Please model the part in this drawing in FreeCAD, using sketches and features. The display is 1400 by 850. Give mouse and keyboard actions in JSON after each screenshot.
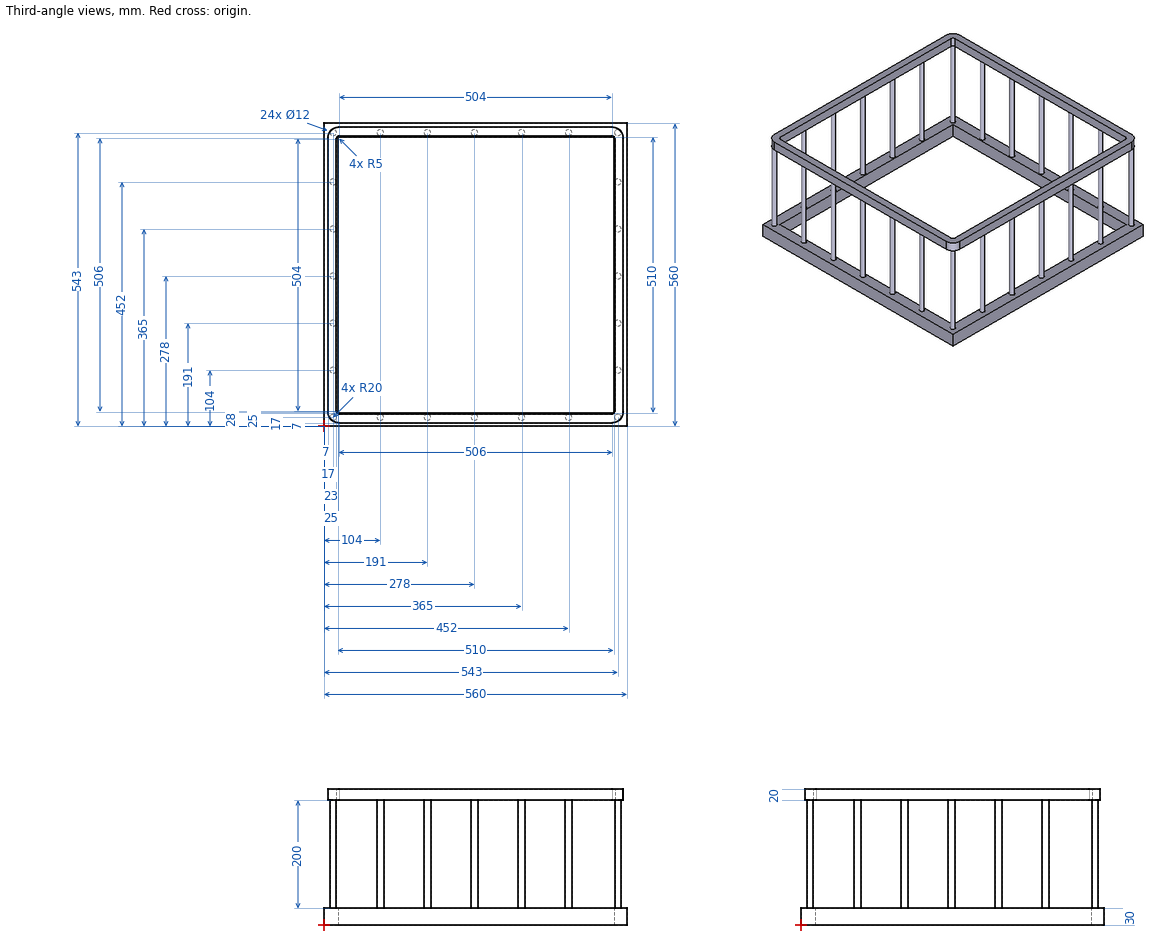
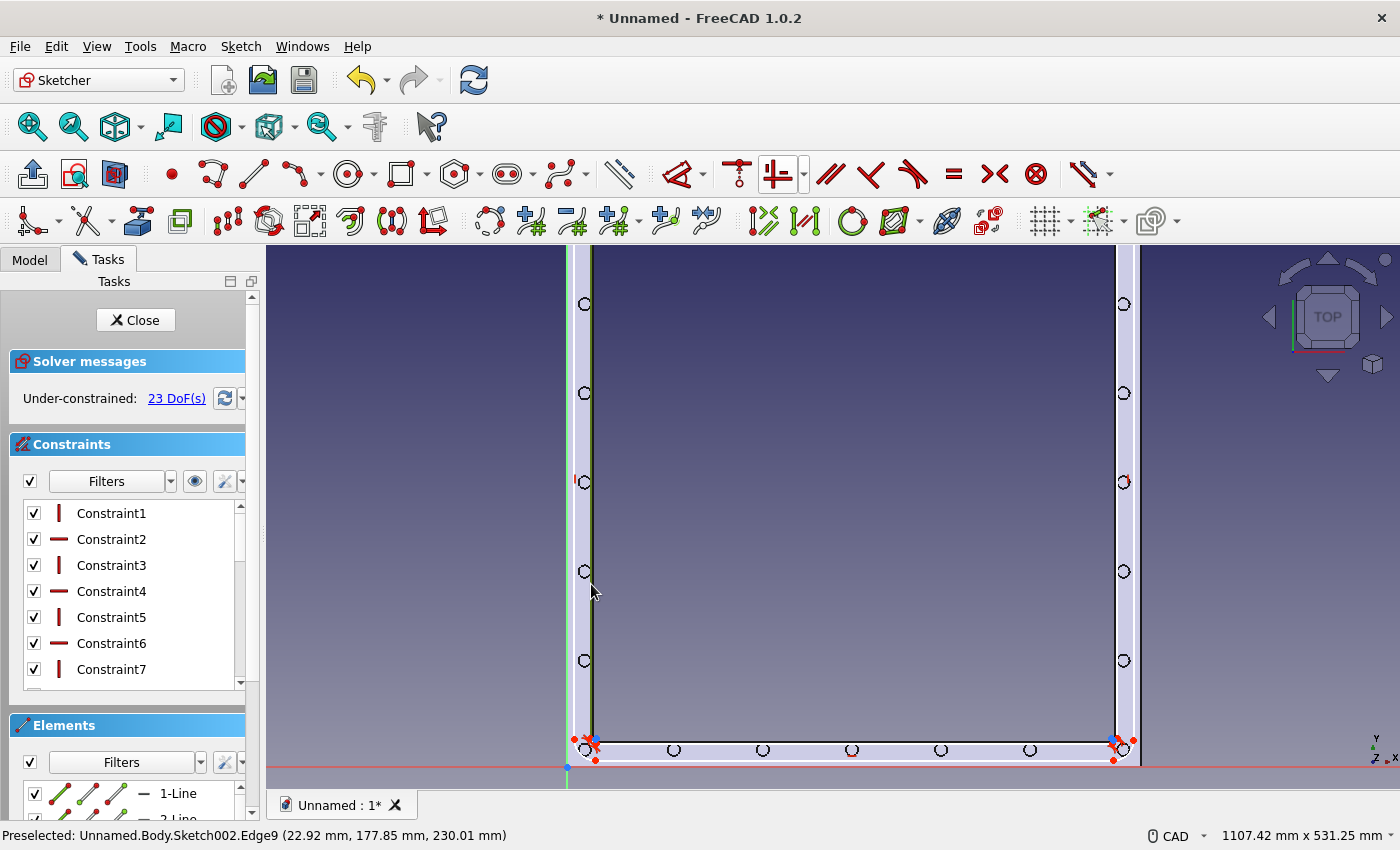
{"action": "scroll", "coordinate": [592, 742], "scroll_direction": "up", "scroll_amount": 7}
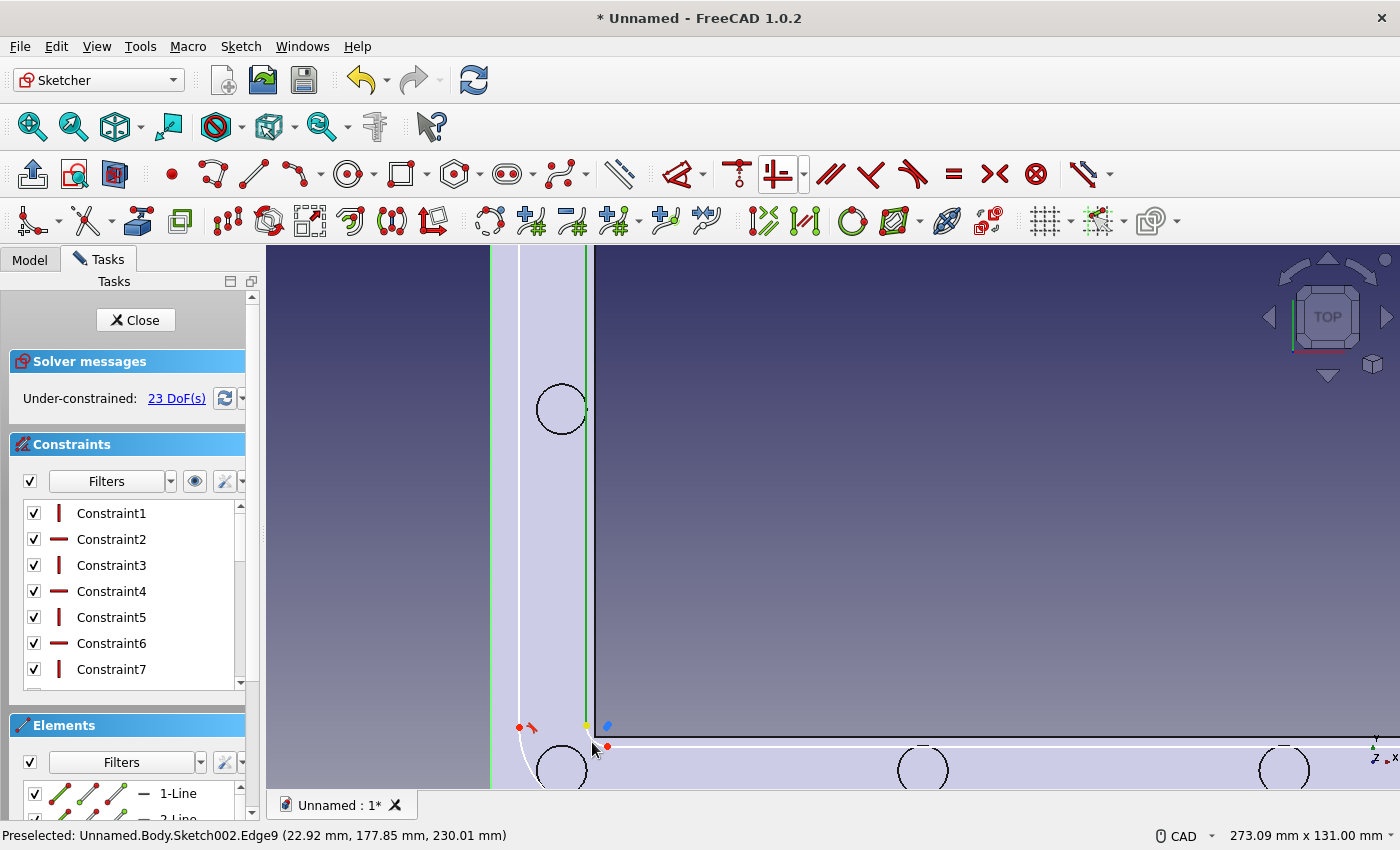
{"action": "left_click", "coordinate": [593, 740]}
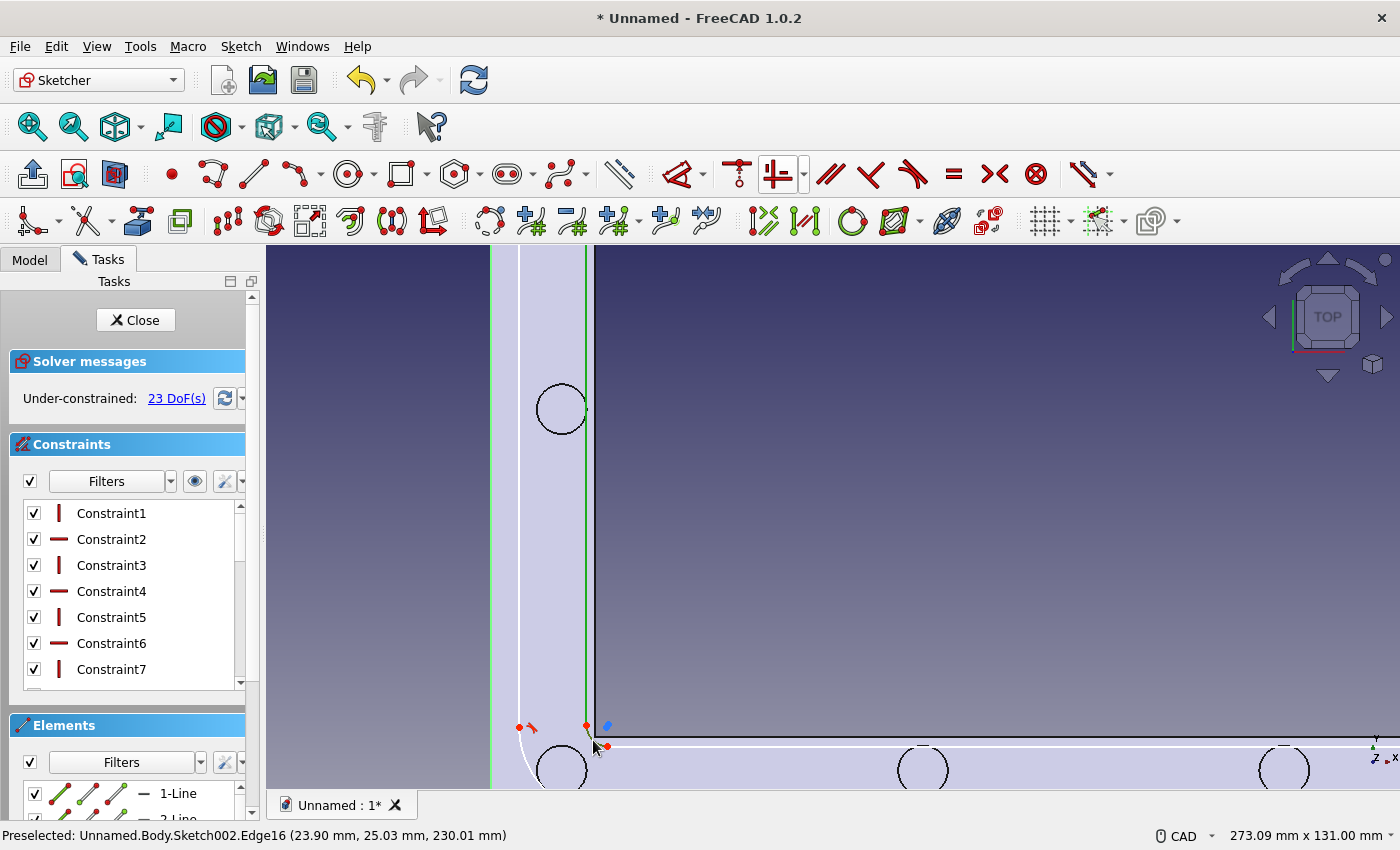
{"action": "left_click", "coordinate": [913, 174]}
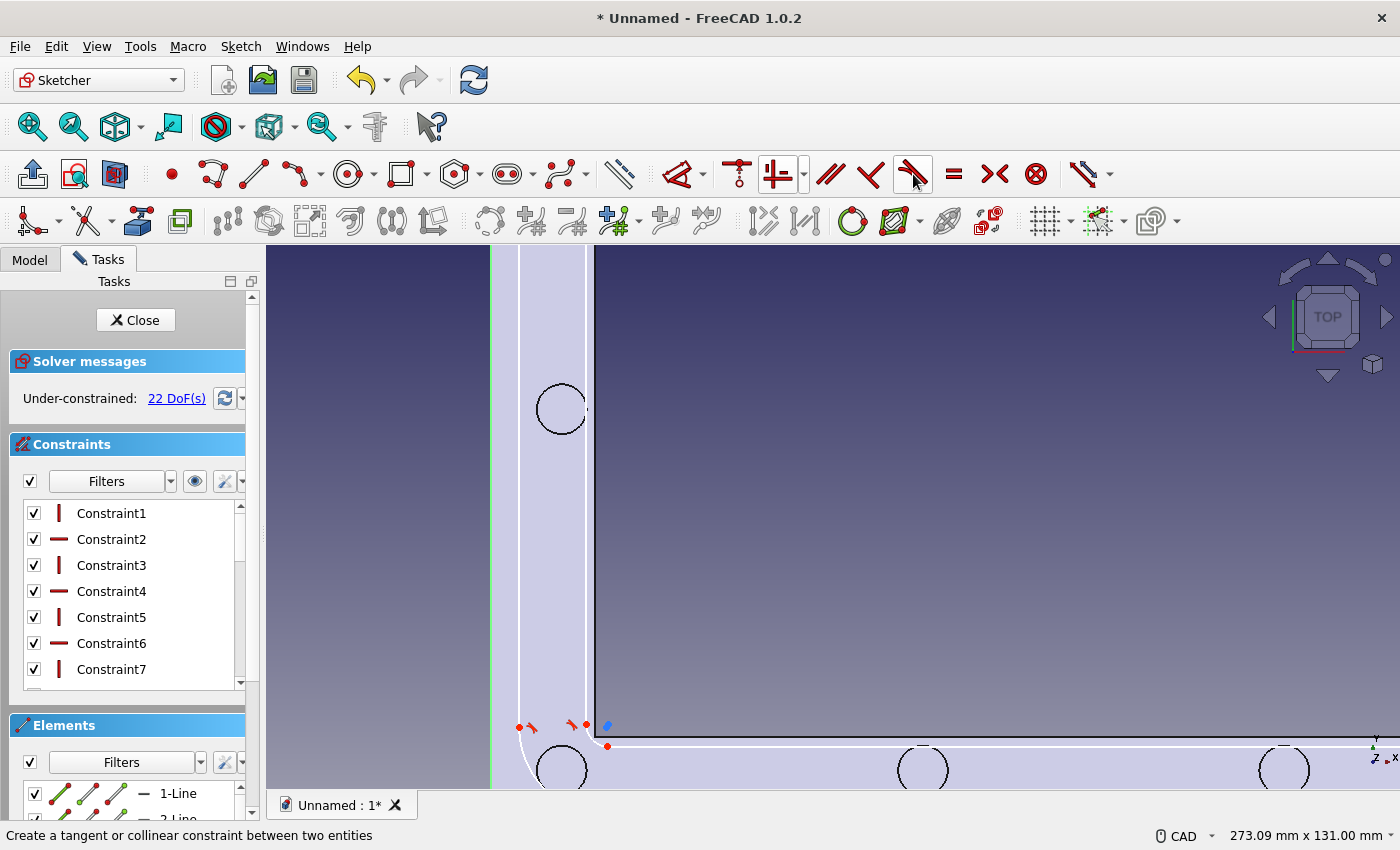
{"action": "scroll", "coordinate": [591, 680], "scroll_direction": "down", "scroll_amount": 9}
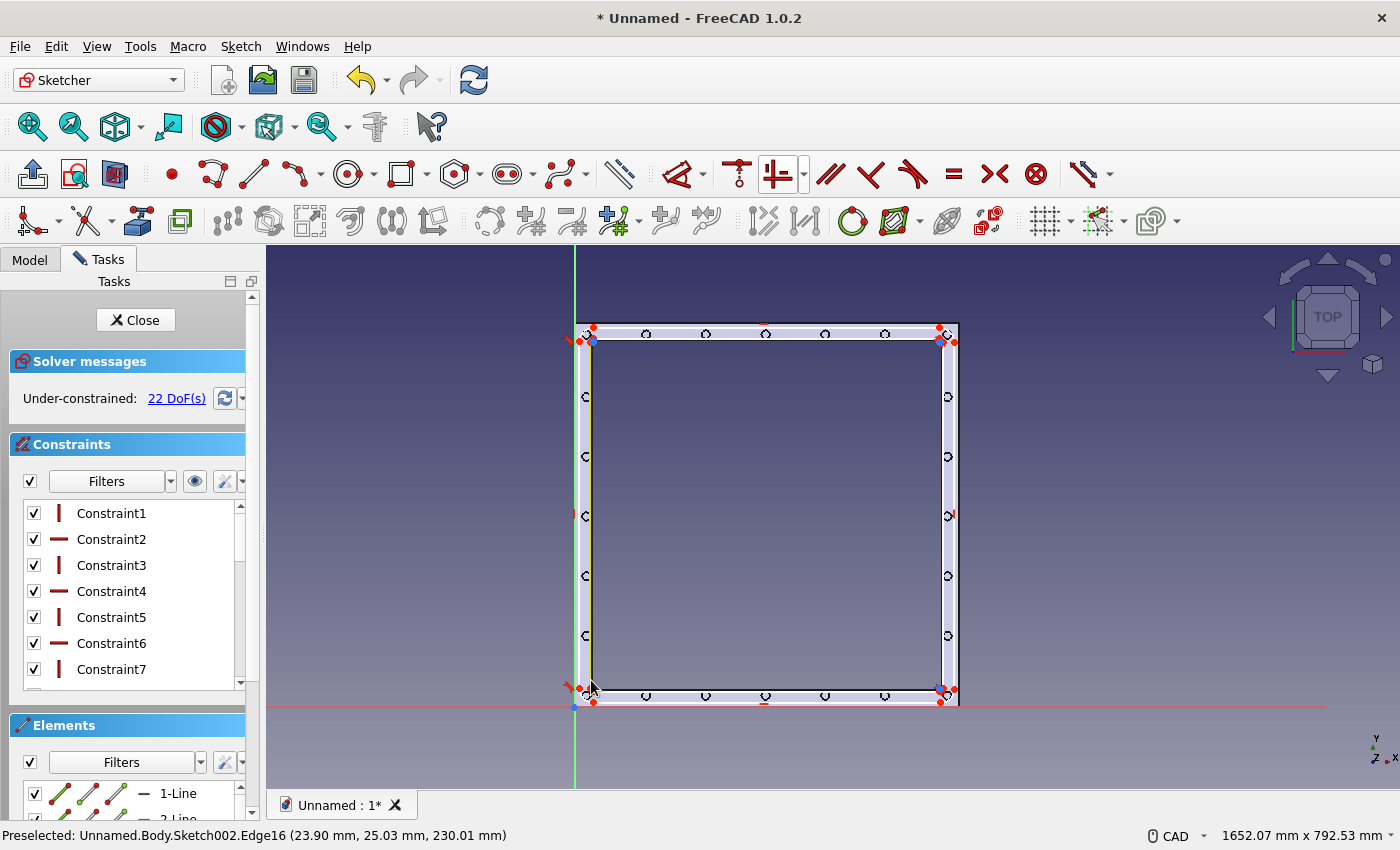
{"action": "scroll", "coordinate": [698, 339], "scroll_direction": "up", "scroll_amount": 2}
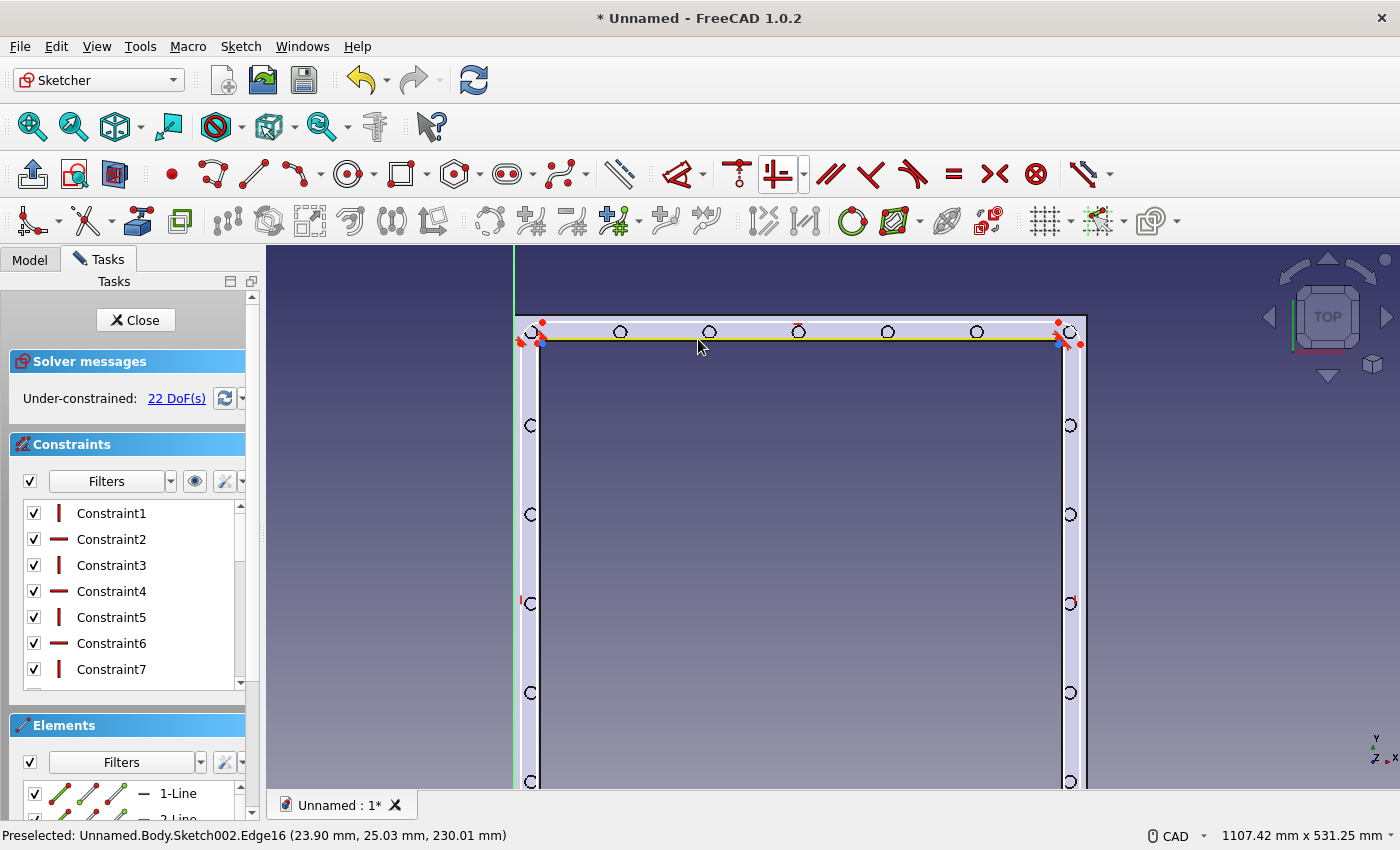
{"action": "left_click", "coordinate": [697, 339]}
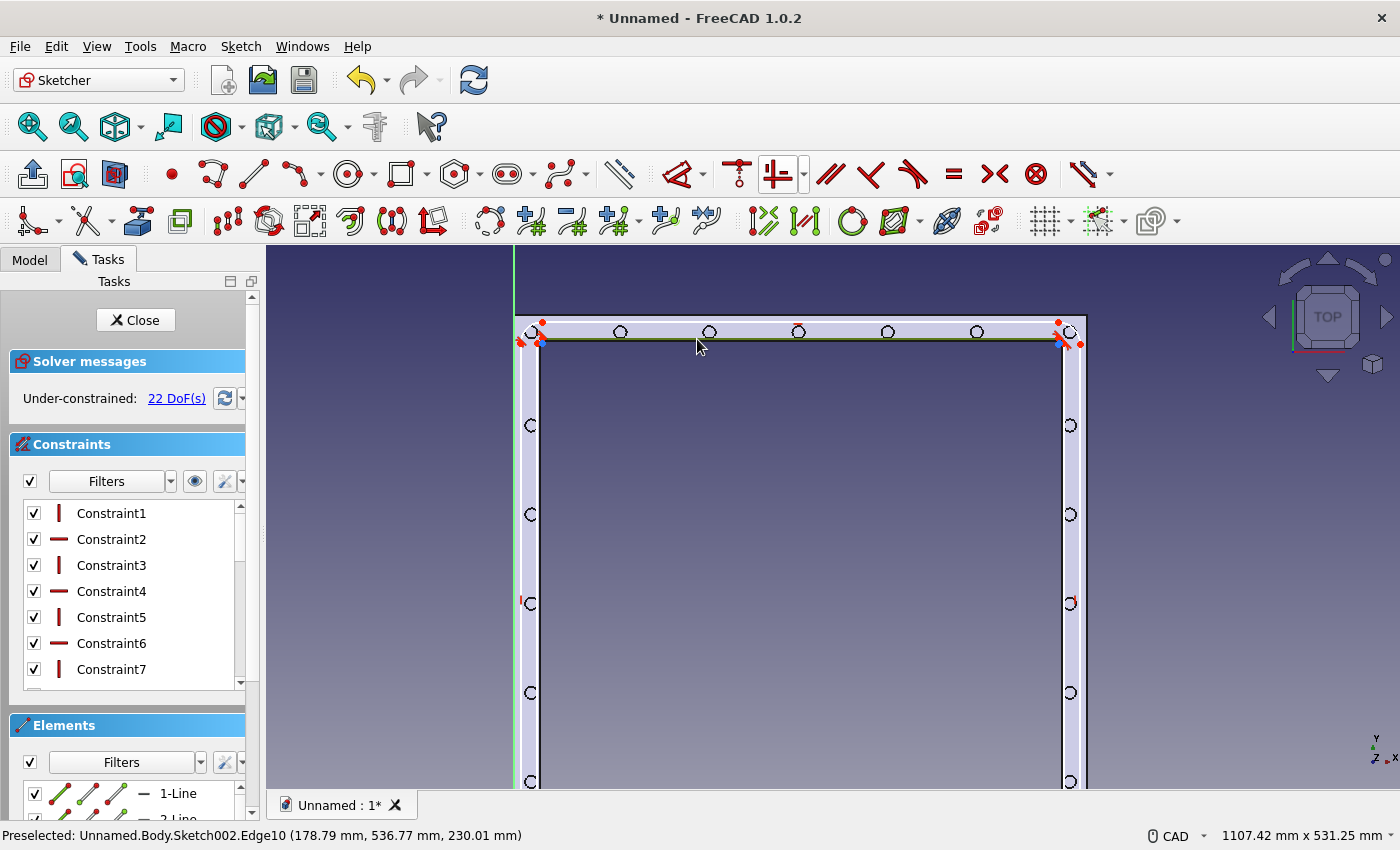
{"action": "scroll", "coordinate": [539, 340], "scroll_direction": "up", "scroll_amount": 7}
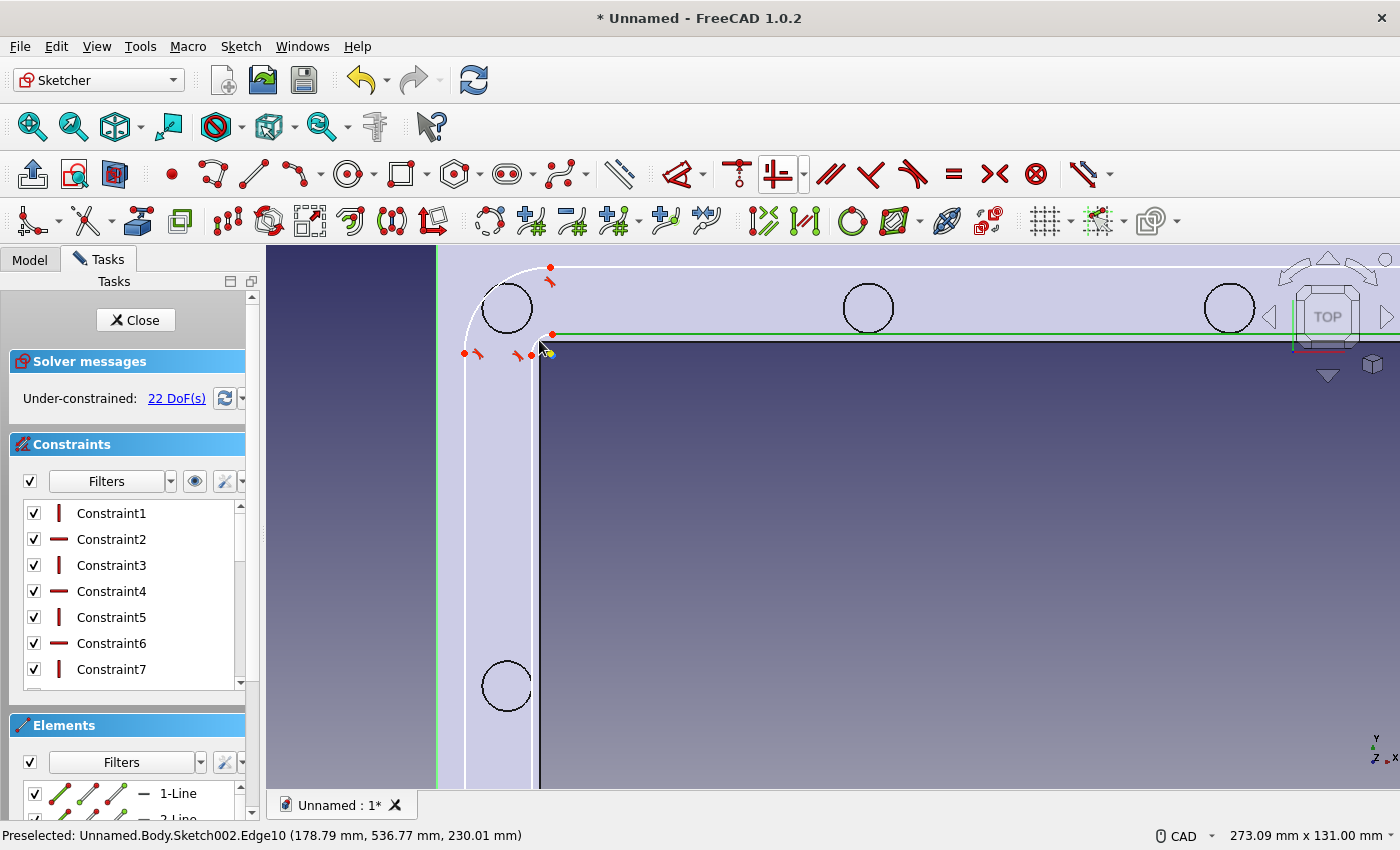
{"action": "left_click", "coordinate": [538, 340]}